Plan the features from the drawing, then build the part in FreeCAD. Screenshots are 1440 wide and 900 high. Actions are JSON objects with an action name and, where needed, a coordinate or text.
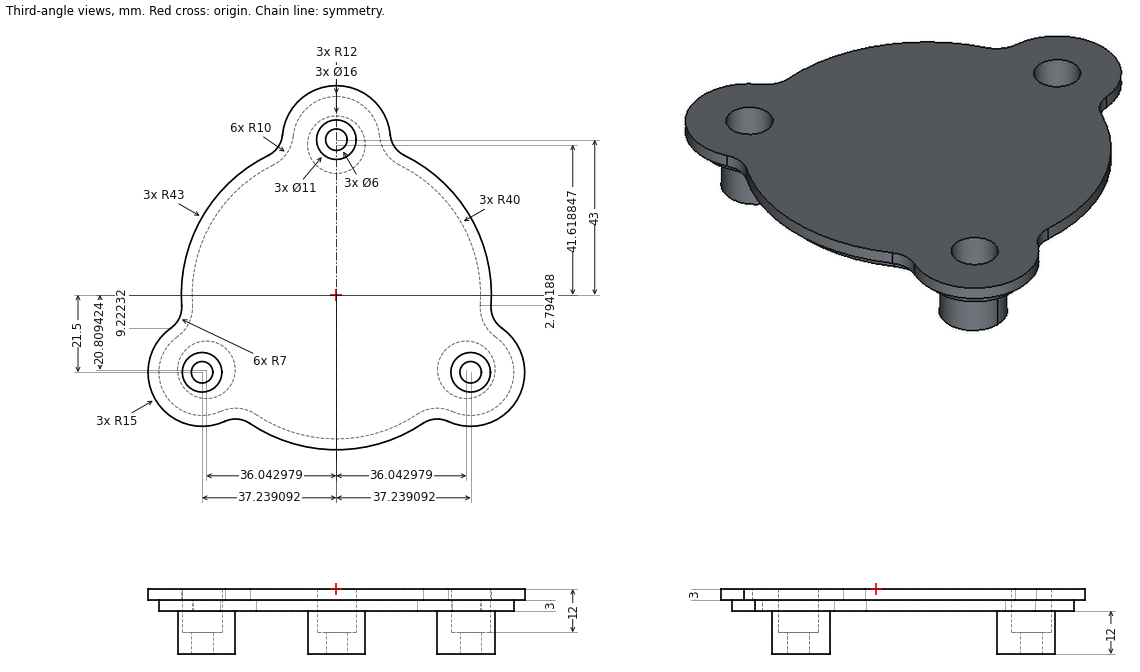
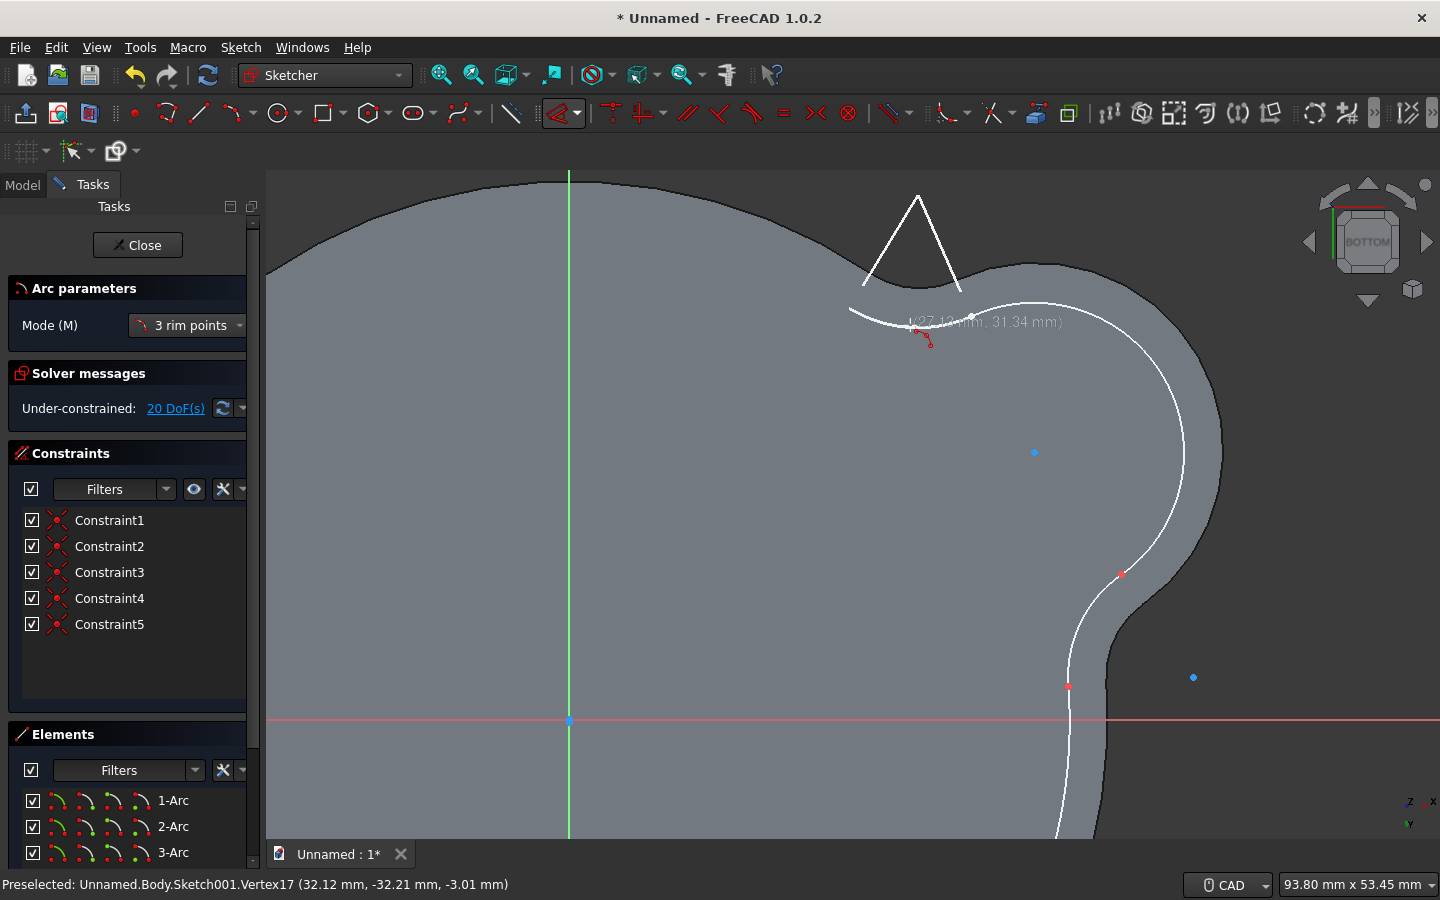
{"action": "left_click", "coordinate": [910, 326]}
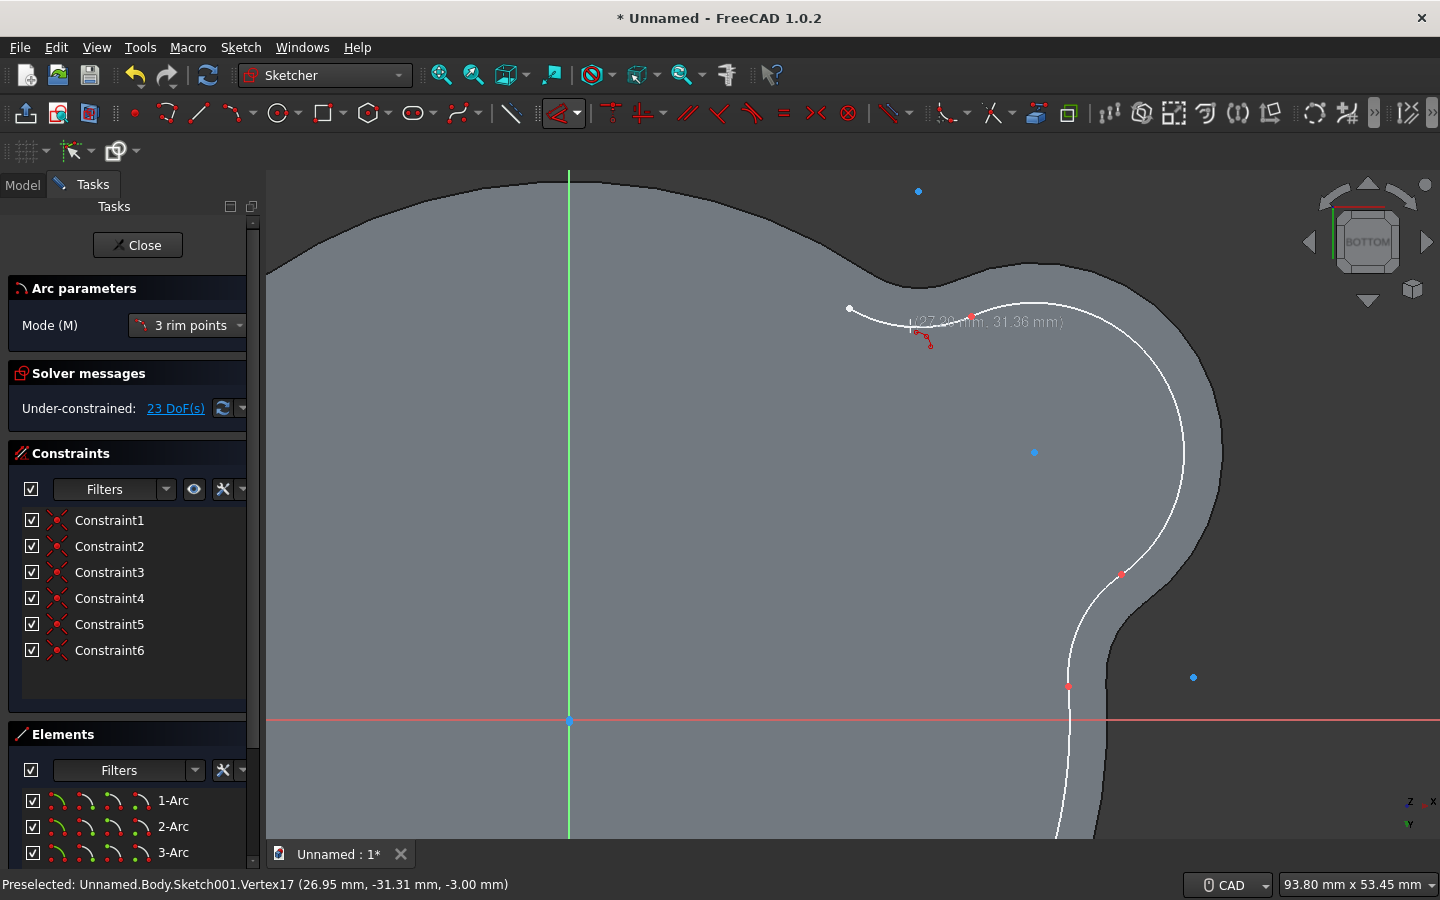
{"action": "left_click", "coordinate": [849, 308]}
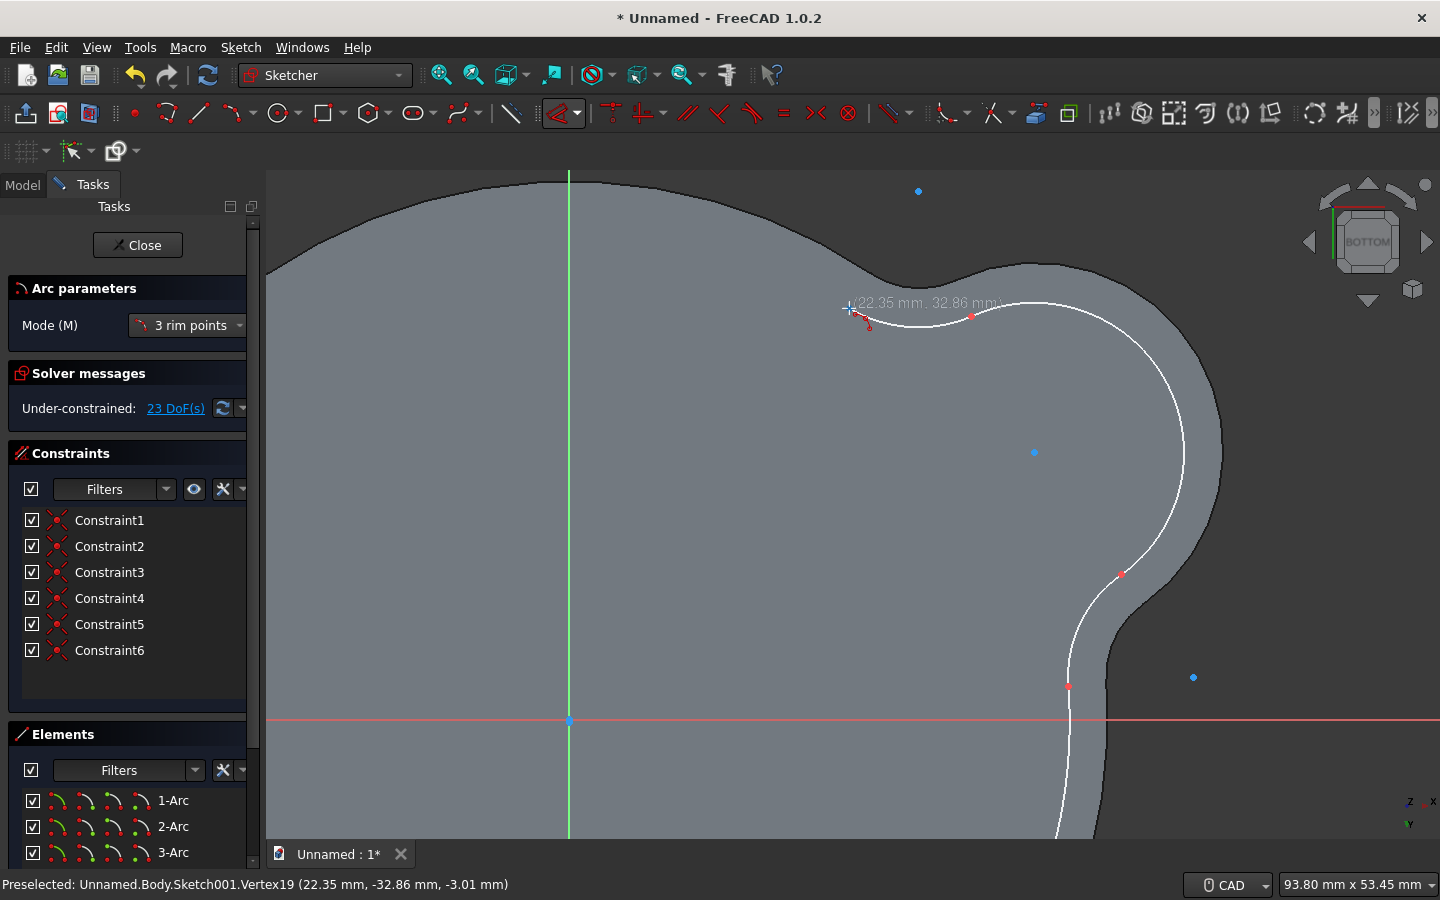
{"action": "scroll", "coordinate": [910, 325], "scroll_direction": "down", "scroll_amount": 5}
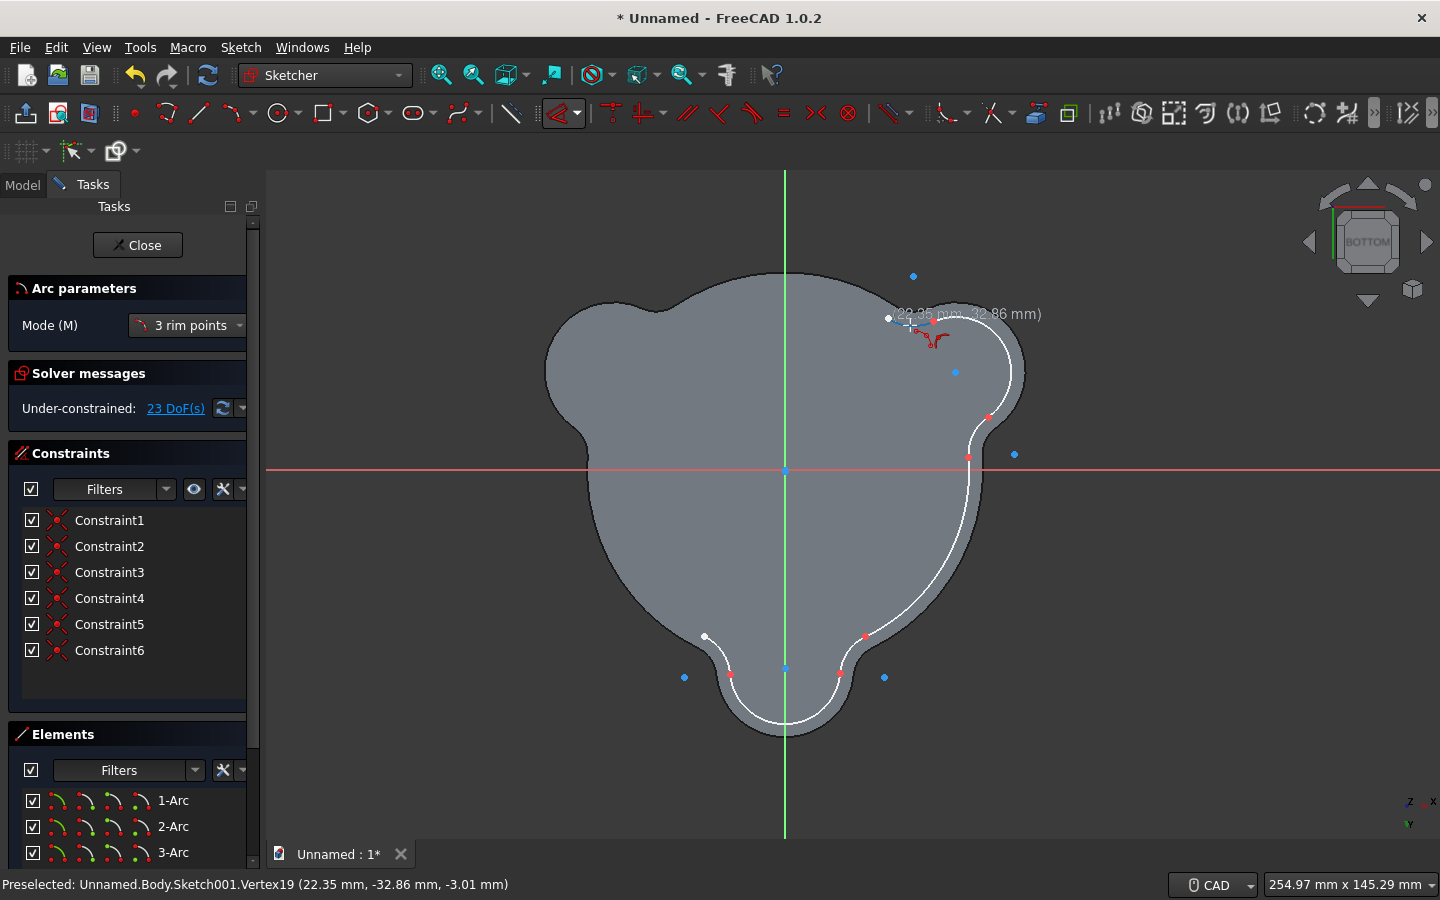
{"action": "left_click", "coordinate": [682, 318]}
{"action": "left_click", "coordinate": [807, 287]}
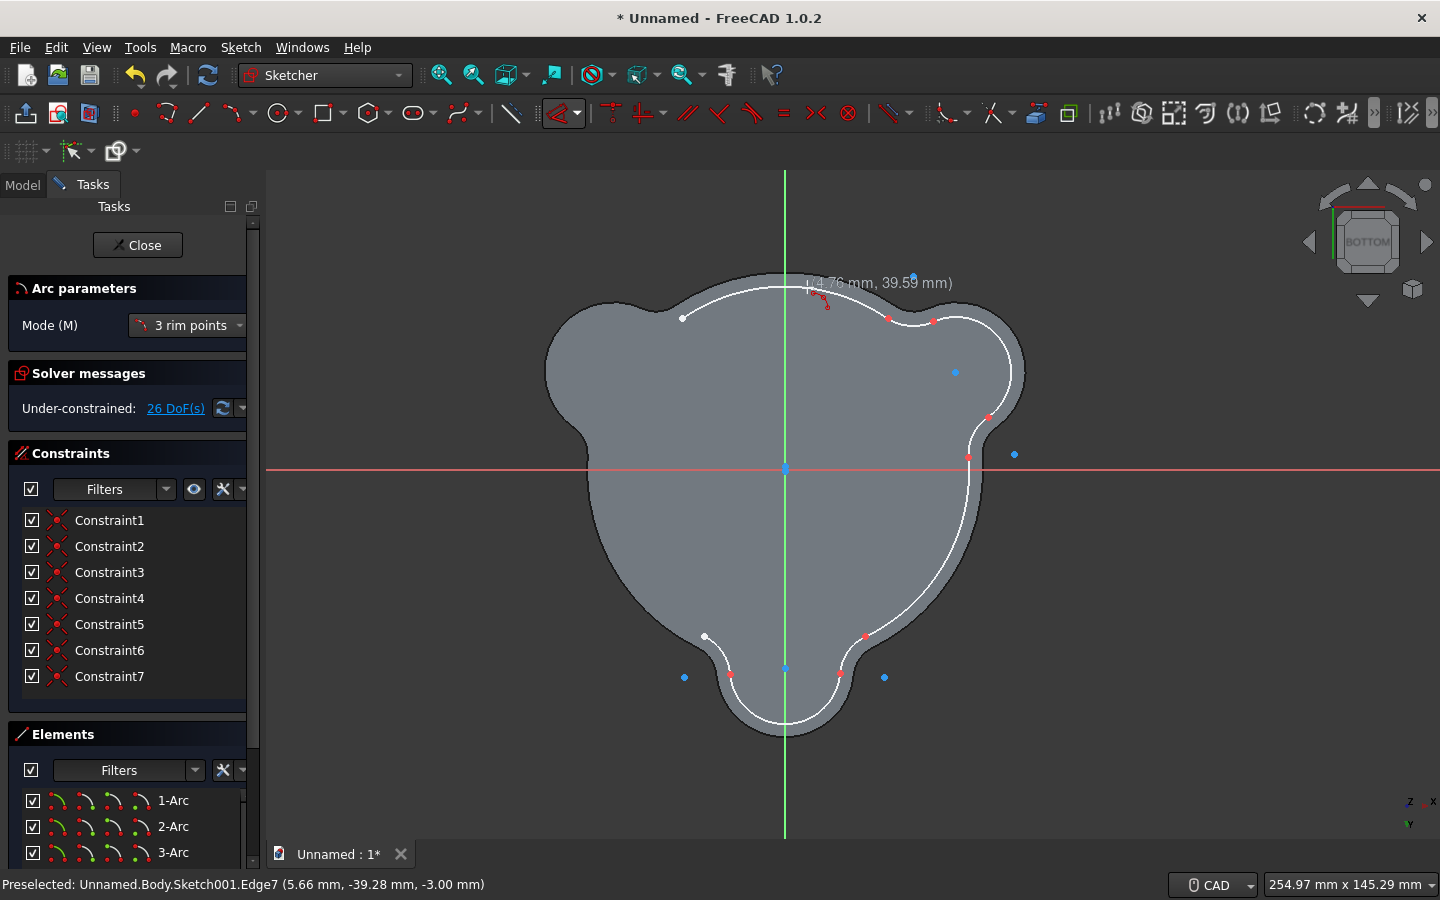
{"action": "left_click", "coordinate": [682, 319]}
{"action": "left_click", "coordinate": [637, 321]}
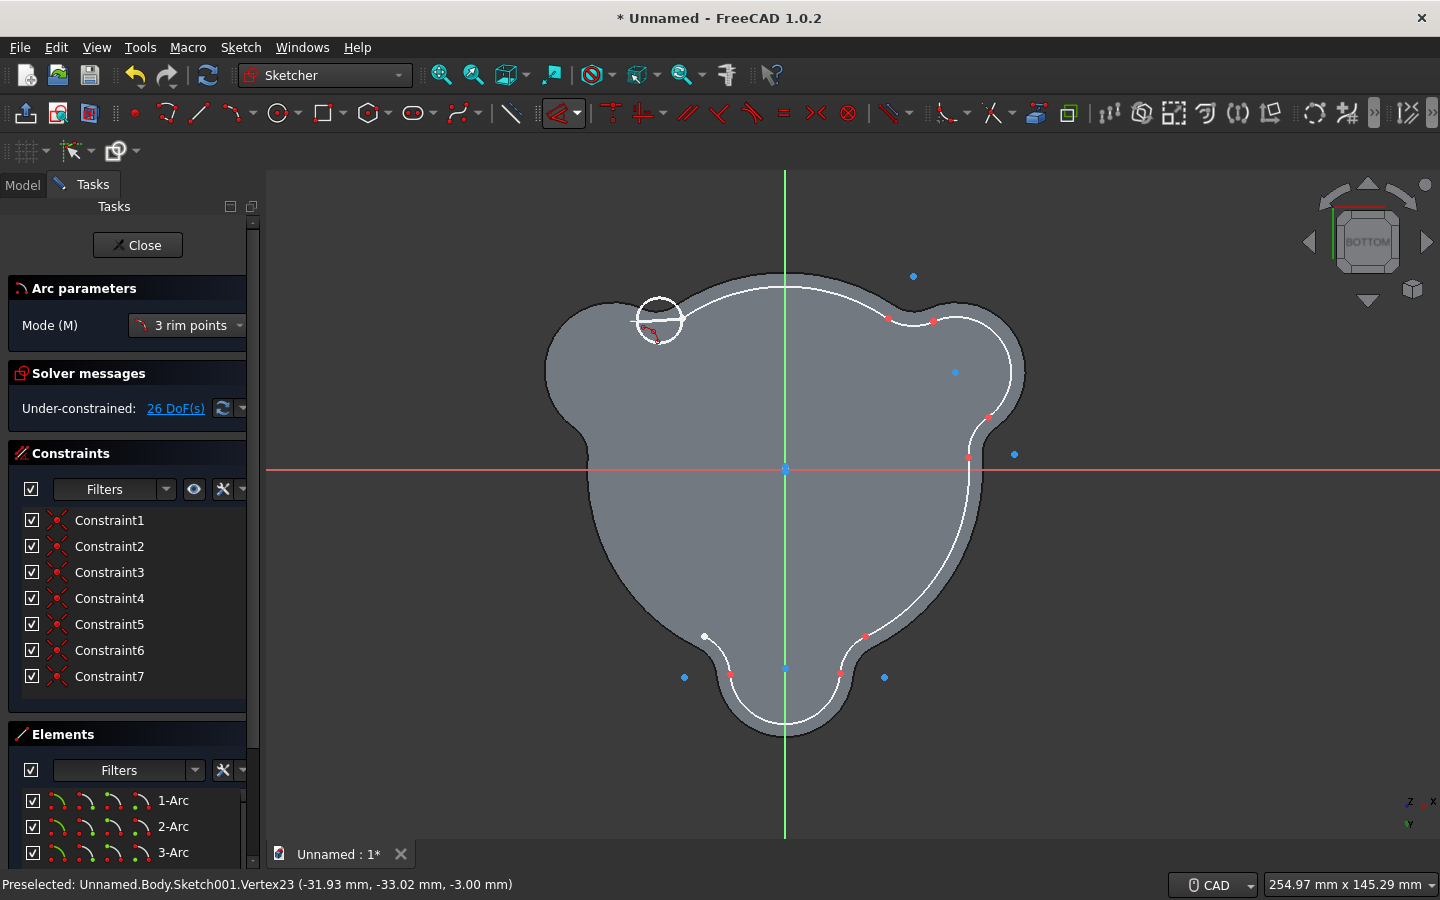
{"action": "scroll", "coordinate": [660, 325], "scroll_direction": "up", "scroll_amount": 5}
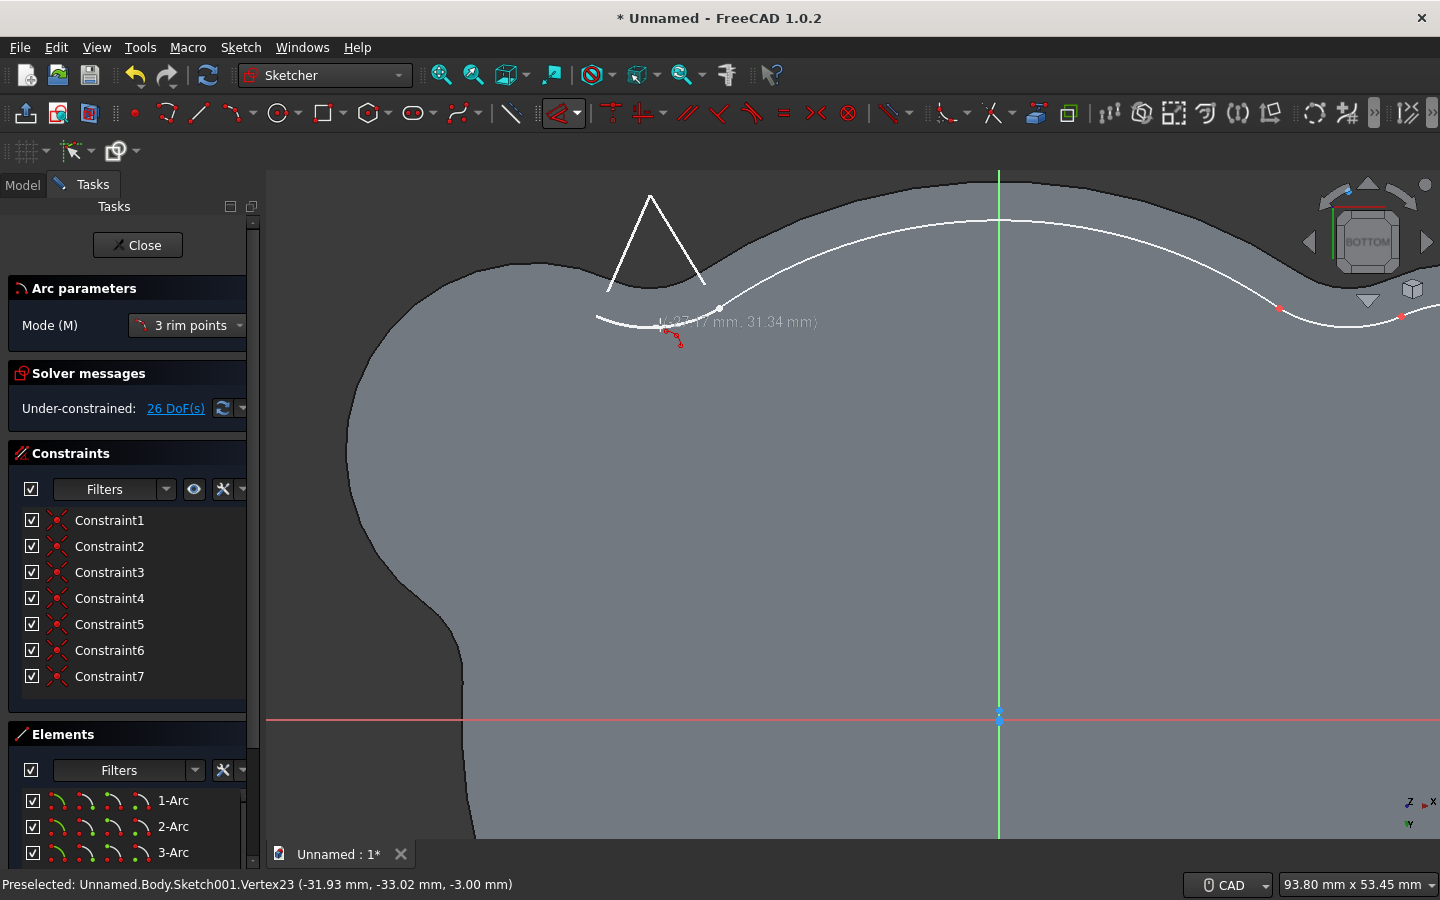
{"action": "left_click", "coordinate": [659, 326]}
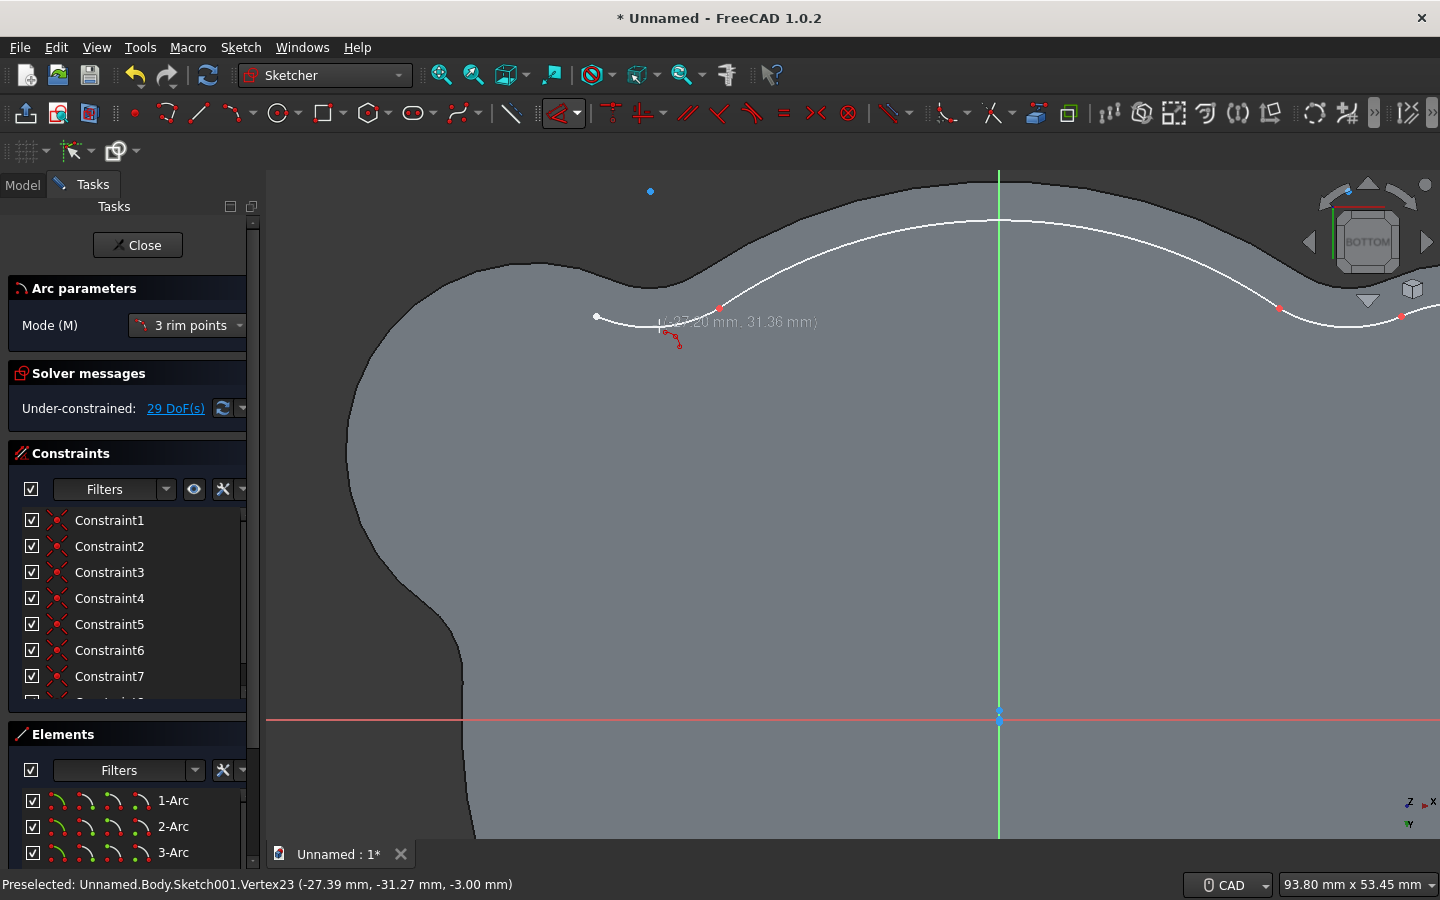
{"action": "left_click", "coordinate": [597, 316]}
{"action": "left_click", "coordinate": [447, 573]}
{"action": "left_click", "coordinate": [403, 375]}